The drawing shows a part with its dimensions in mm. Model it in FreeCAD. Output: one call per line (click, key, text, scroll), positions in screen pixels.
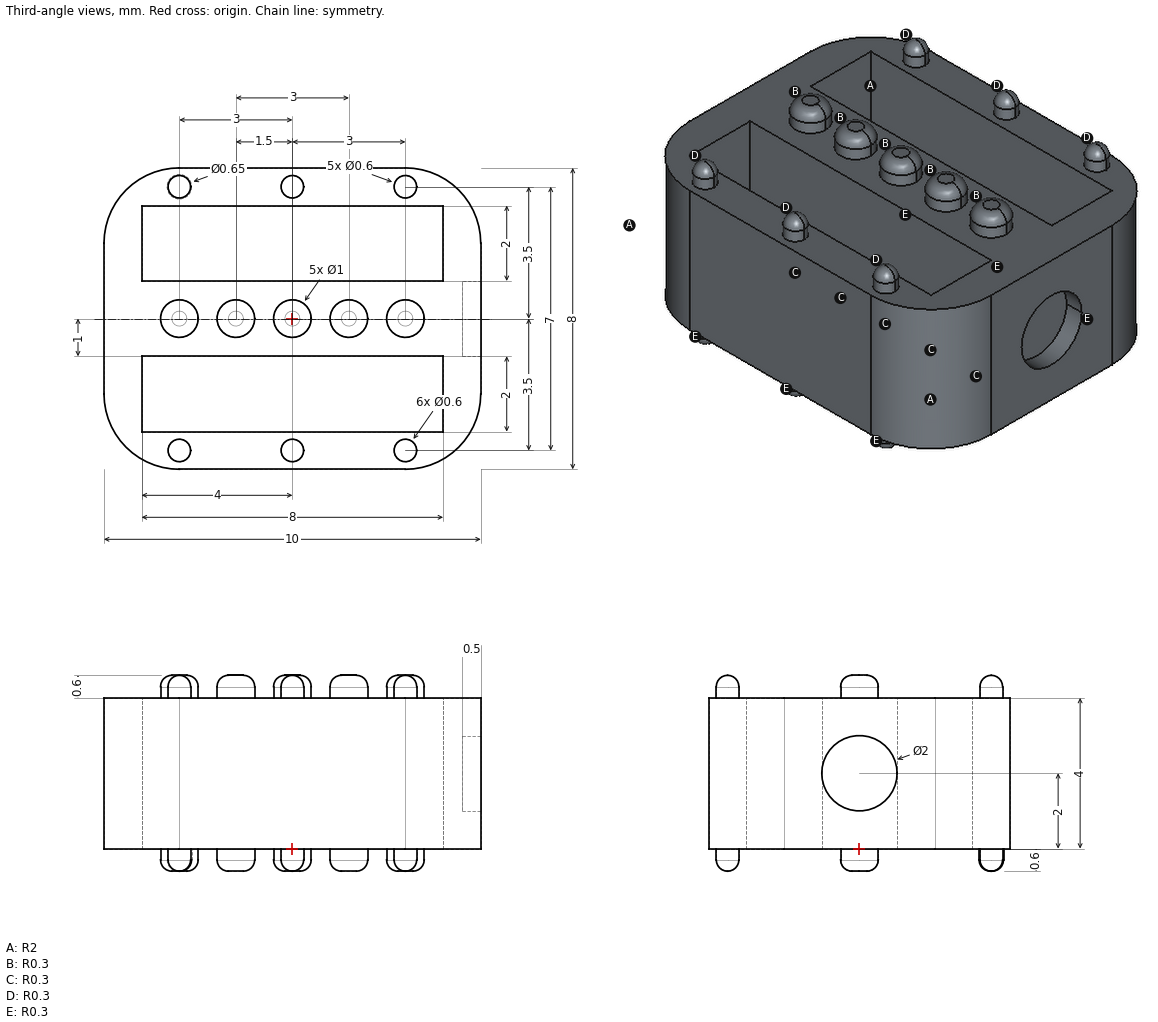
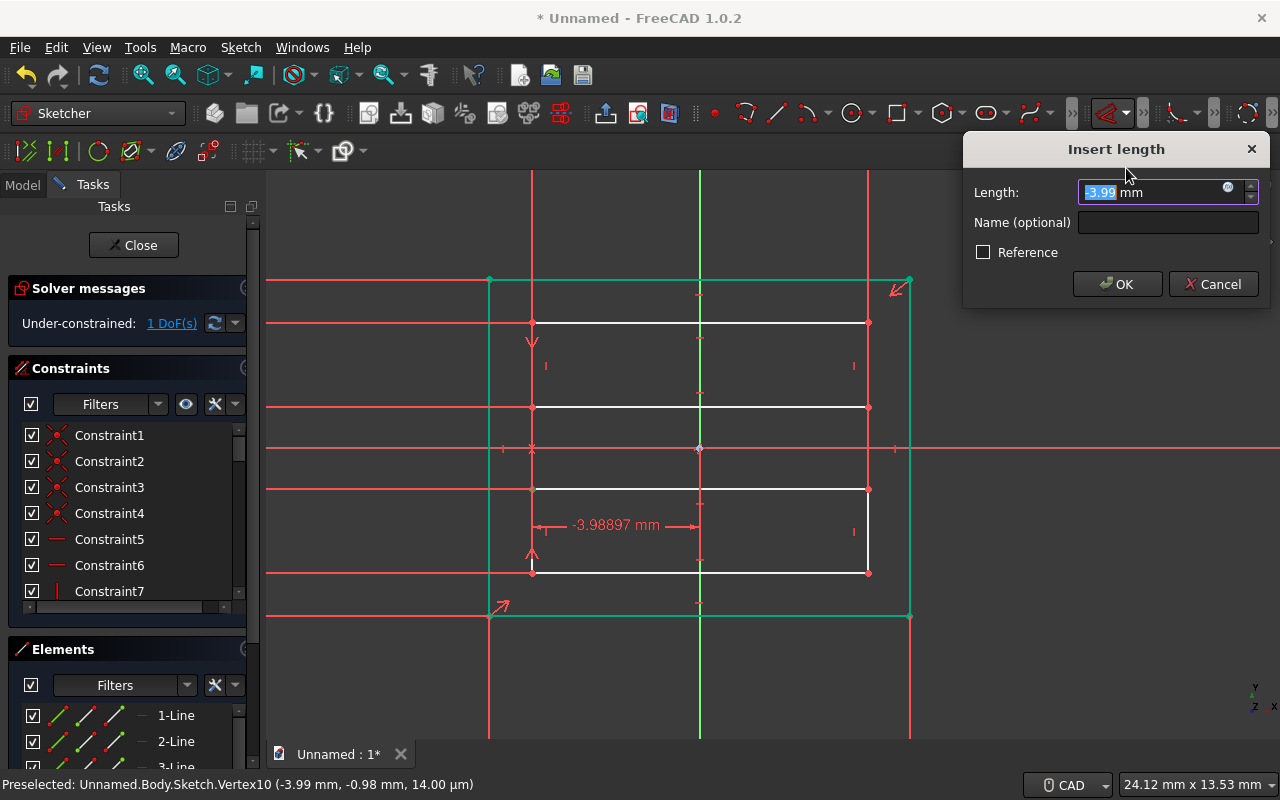
text(-4)
key(Return)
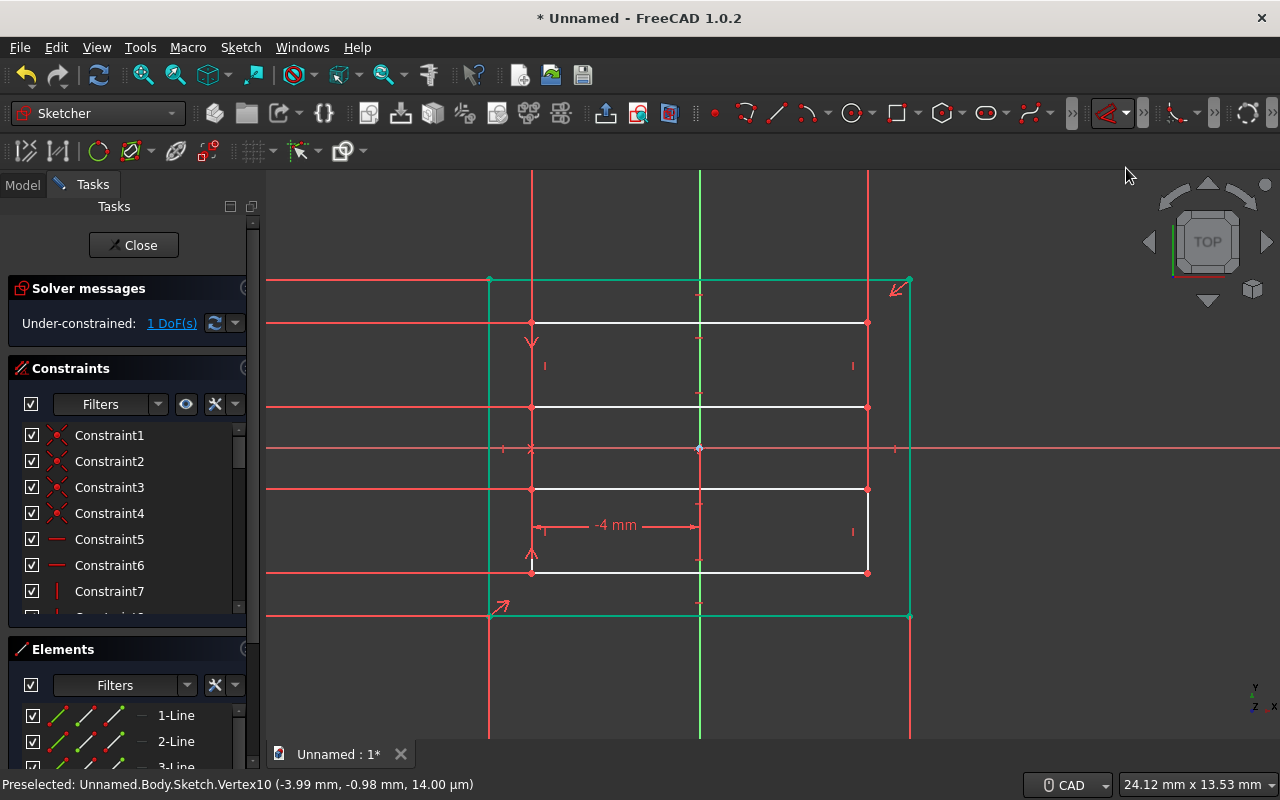
click(532, 489)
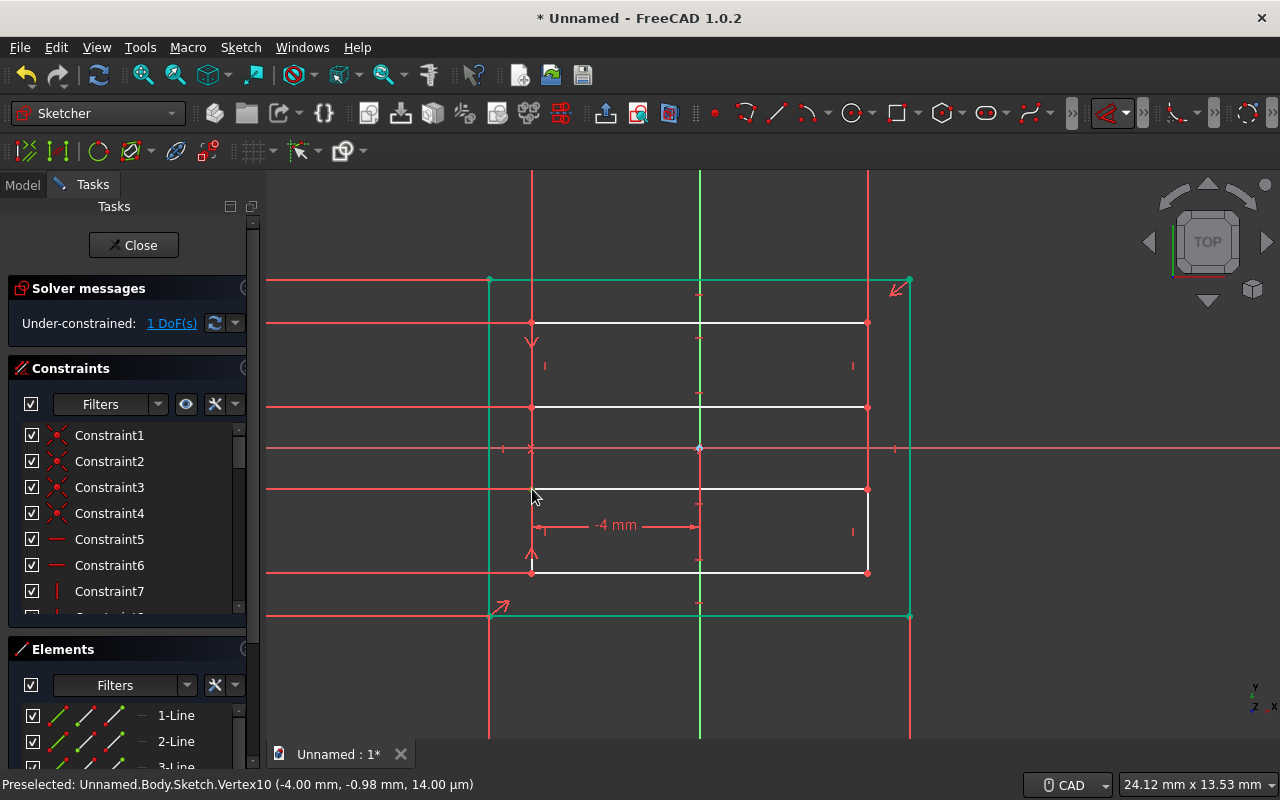
click(1128, 114)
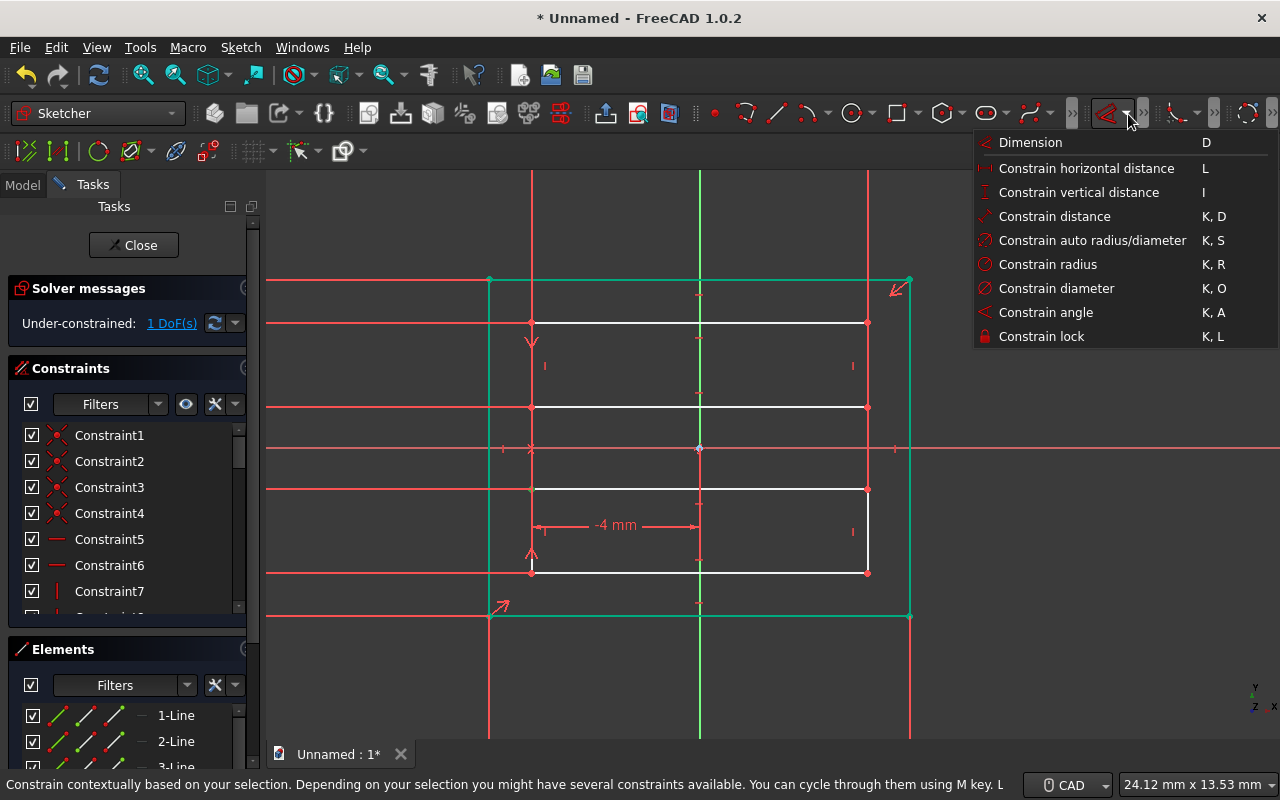
click(1126, 192)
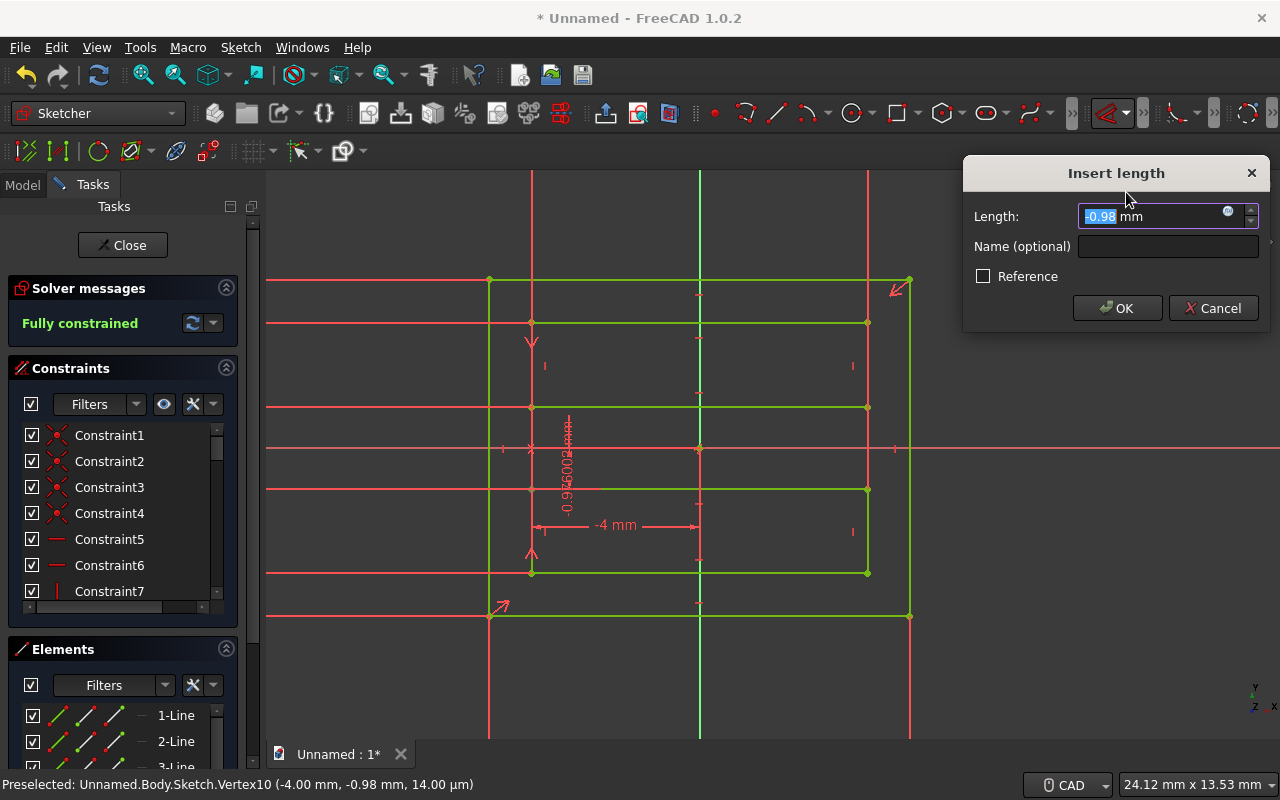
text(-1)
key(Return)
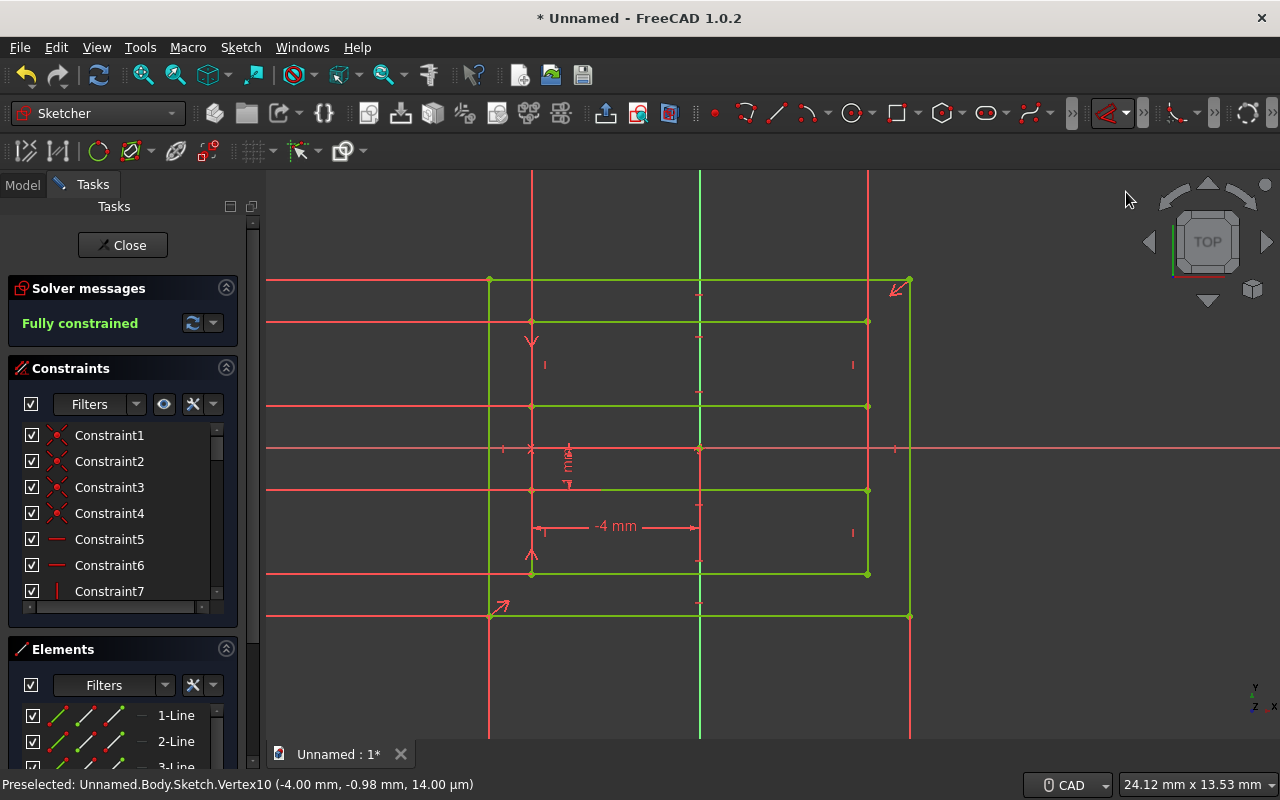
click(123, 245)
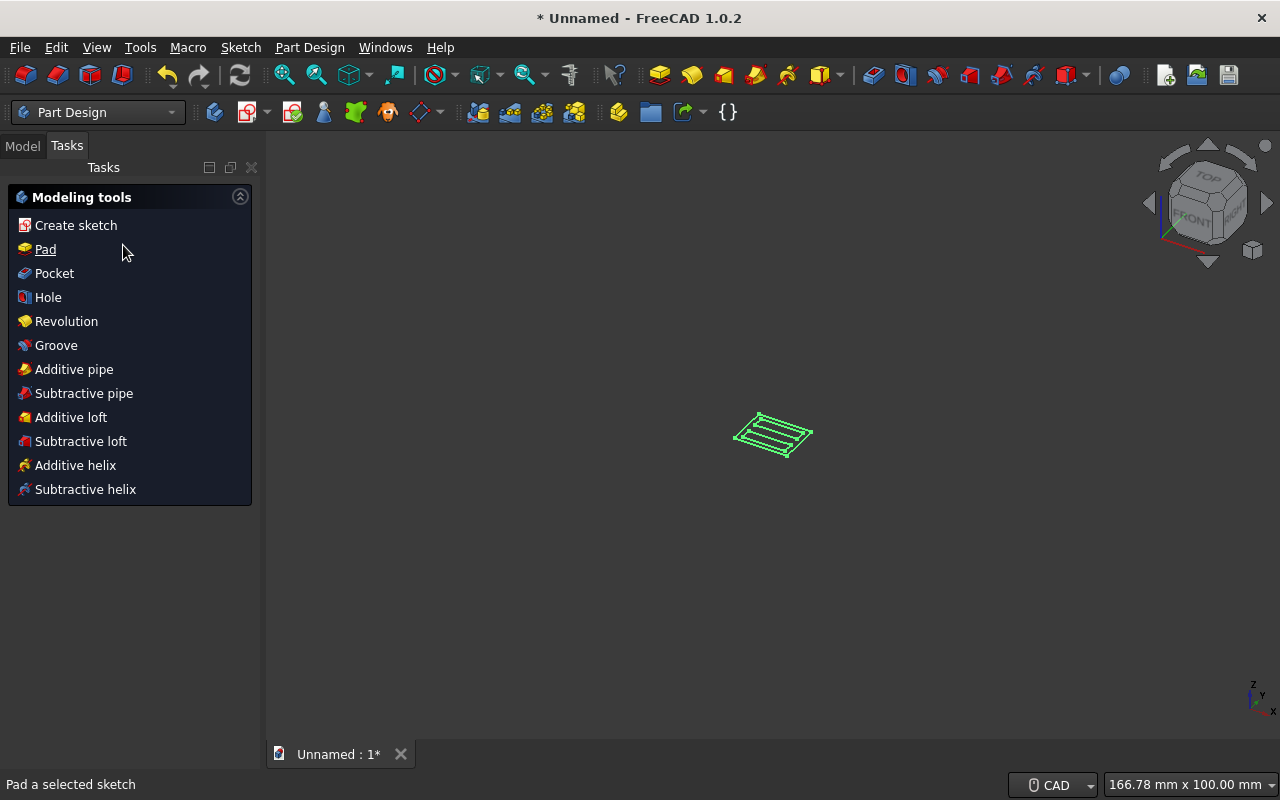
click(660, 76)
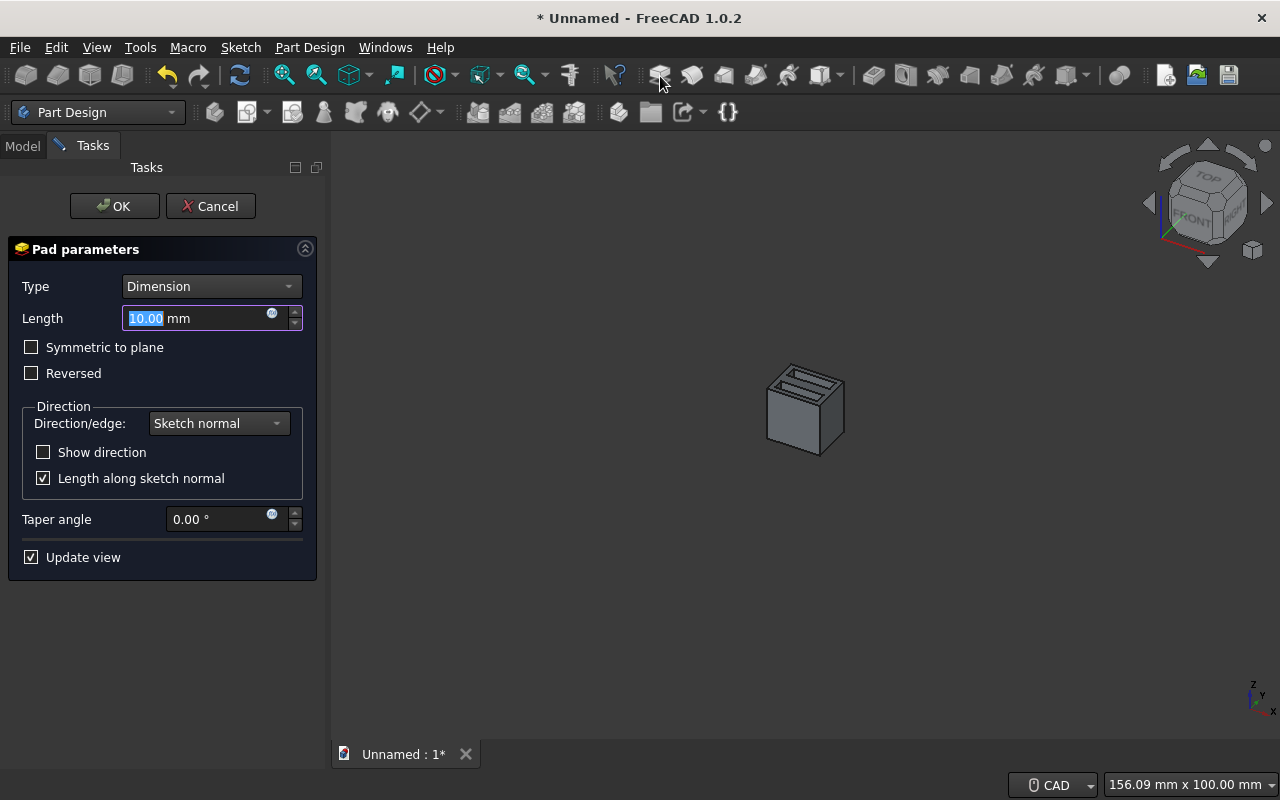
text(4)
key(Tab)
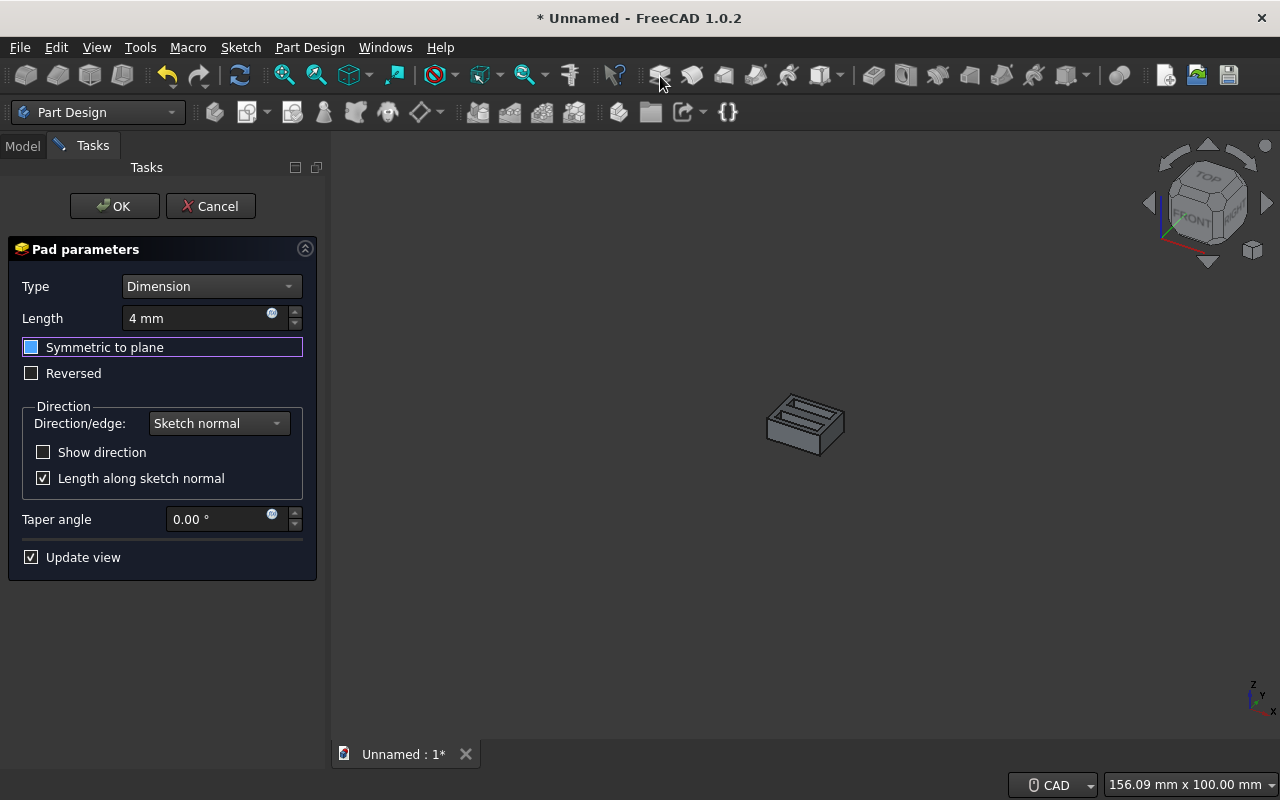
click(115, 206)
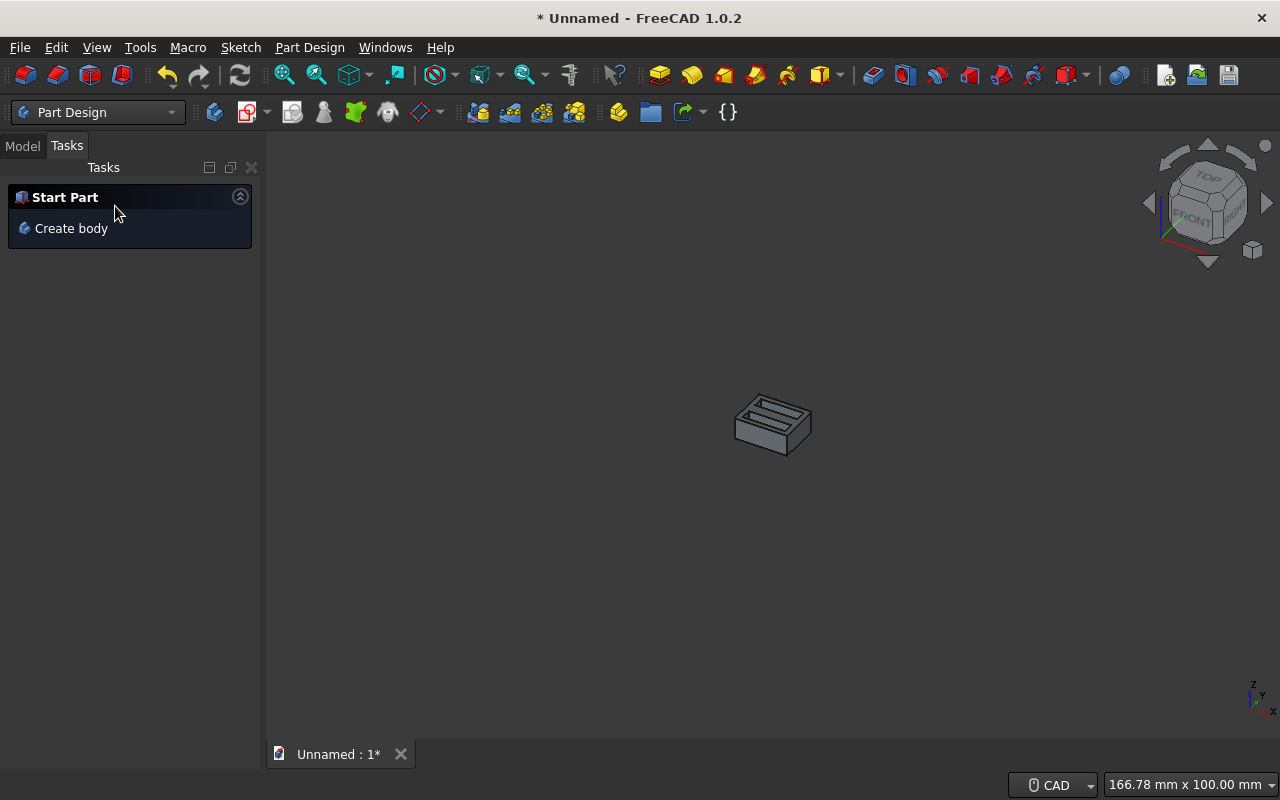
key(v)
key(f)